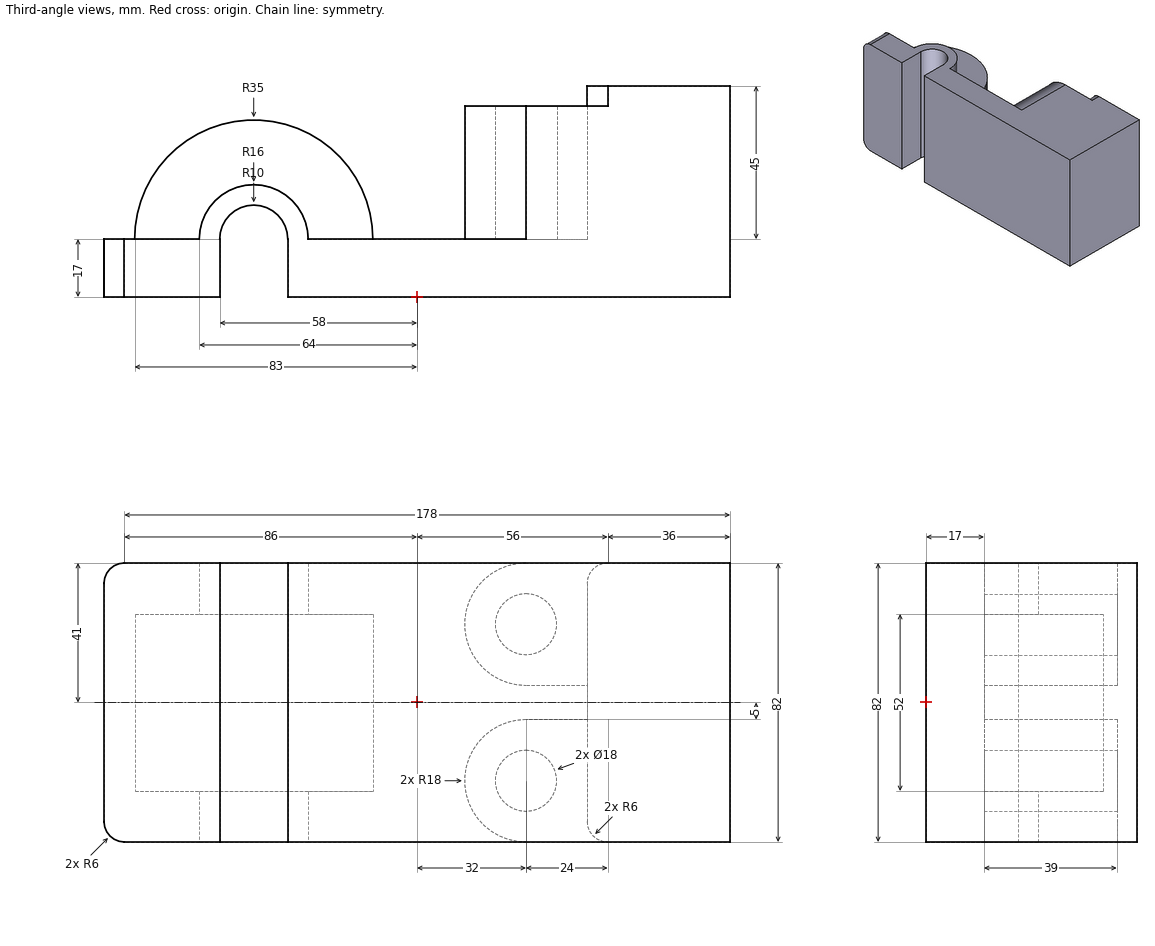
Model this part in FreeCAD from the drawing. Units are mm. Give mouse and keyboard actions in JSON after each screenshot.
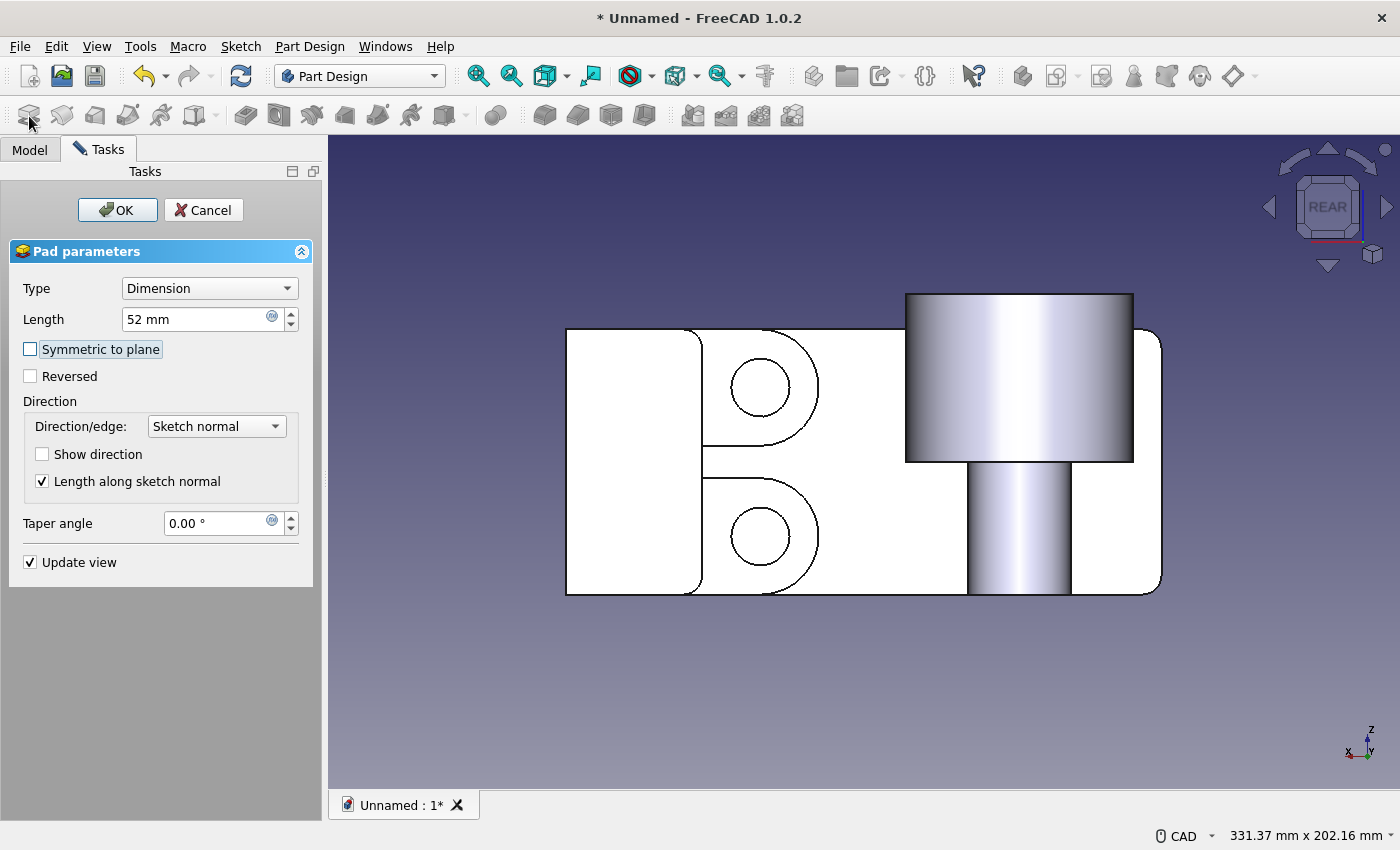
{"action": "left_click", "coordinate": [31, 349]}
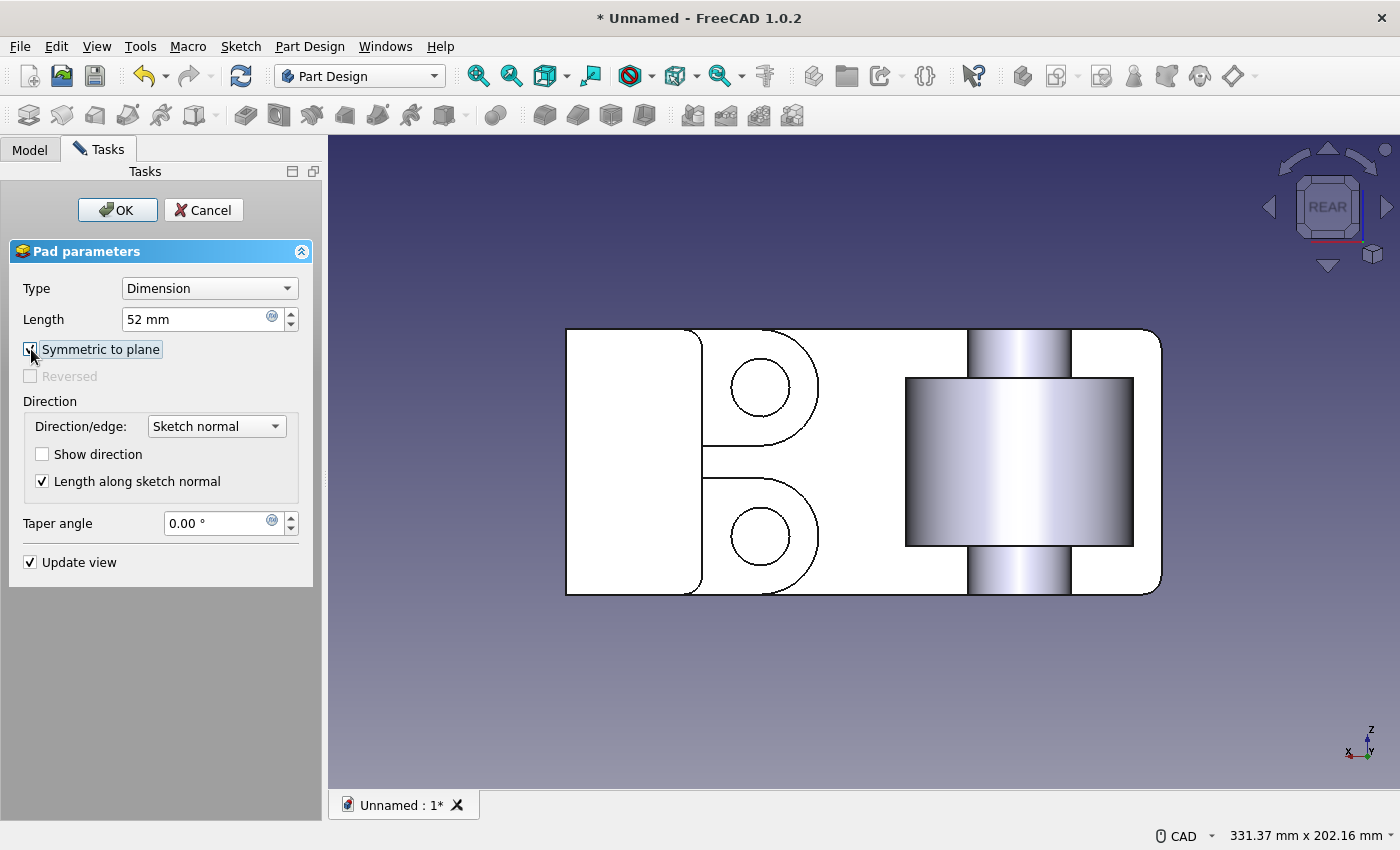
{"action": "left_click", "coordinate": [118, 210]}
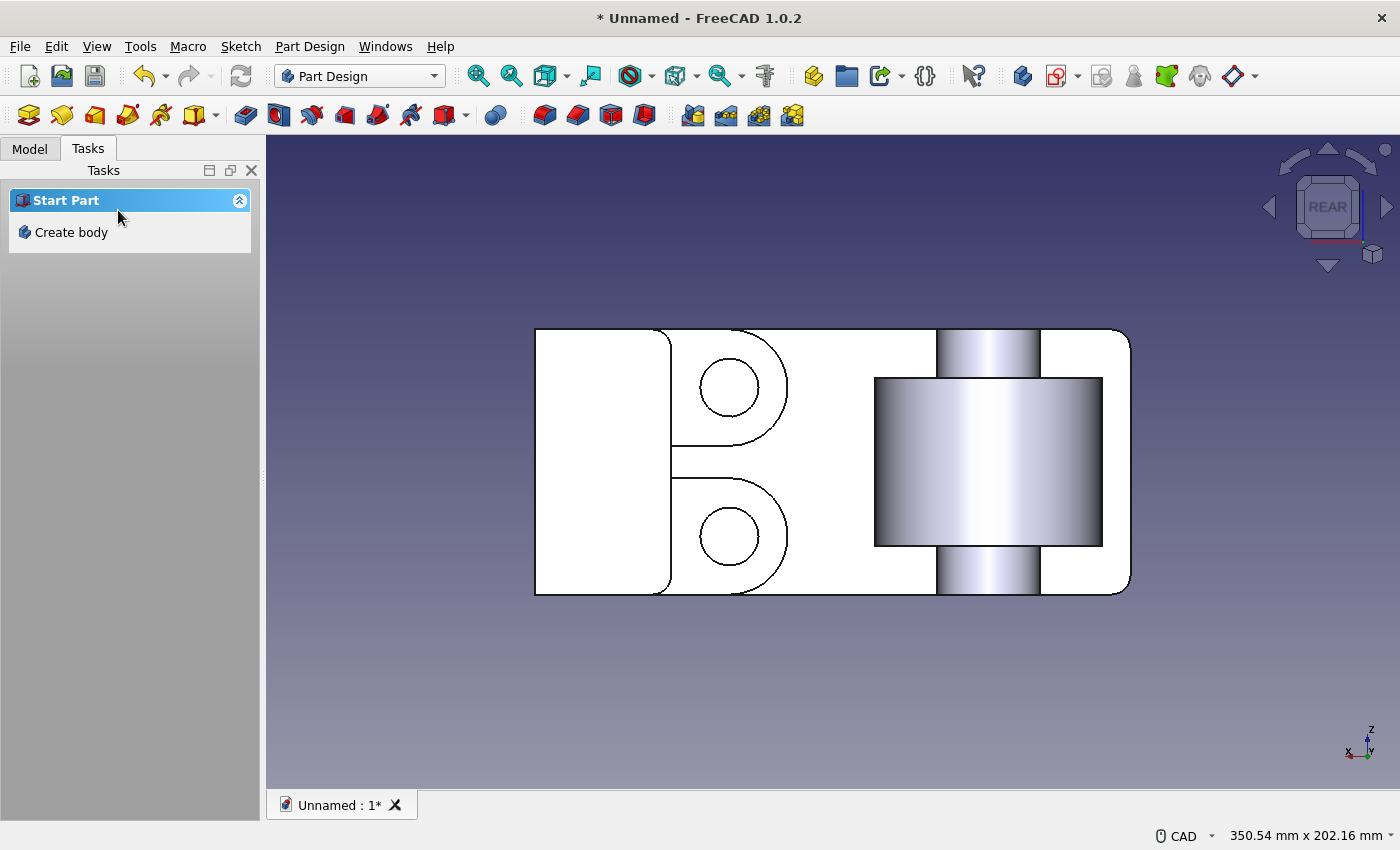
{"action": "key", "text": "0"}